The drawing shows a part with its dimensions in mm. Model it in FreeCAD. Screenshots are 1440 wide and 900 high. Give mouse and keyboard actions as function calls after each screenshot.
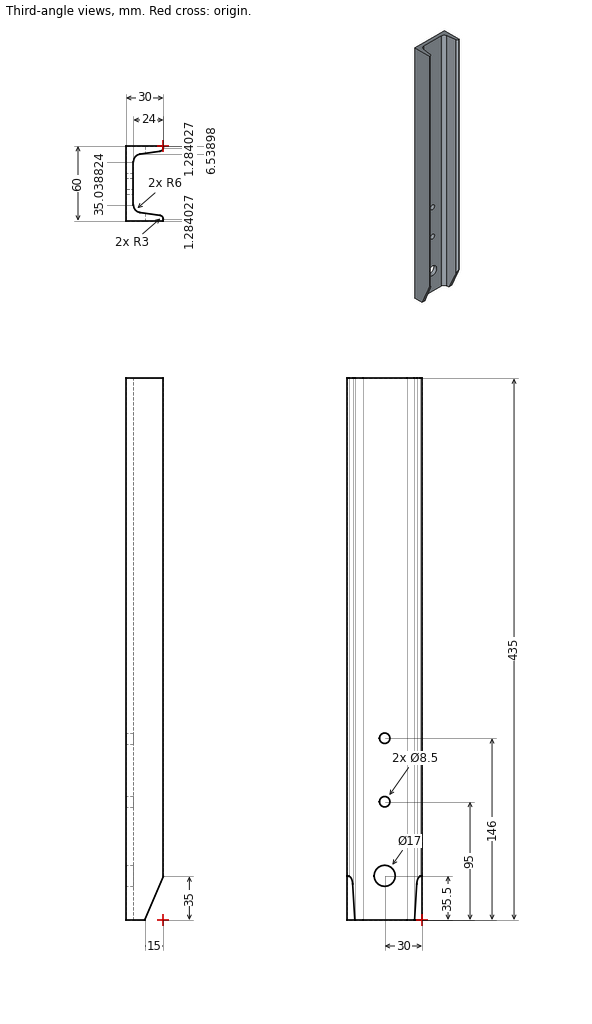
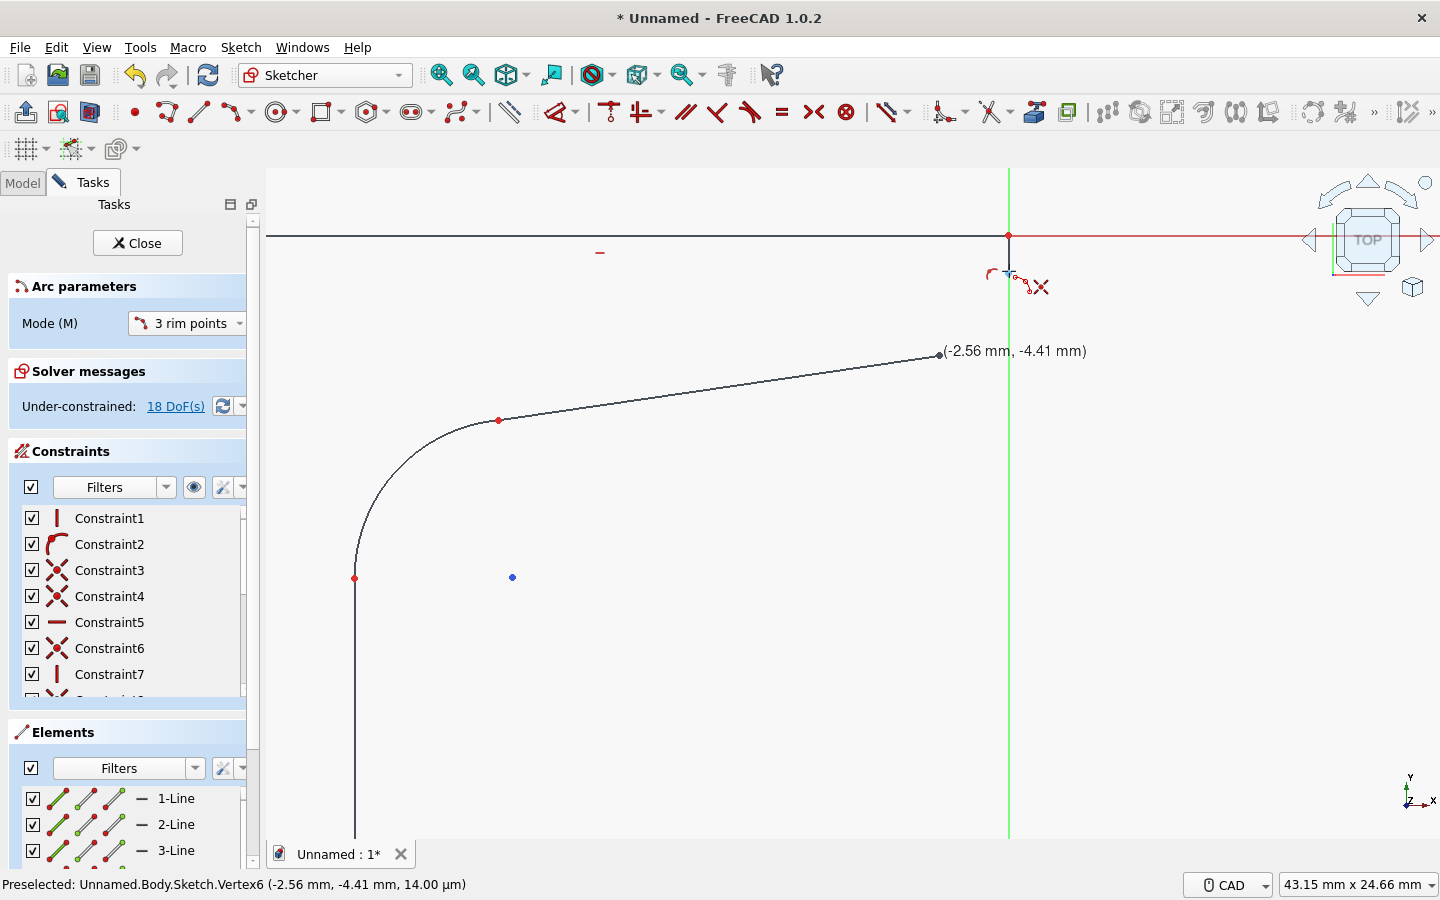
click(1009, 273)
click(989, 324)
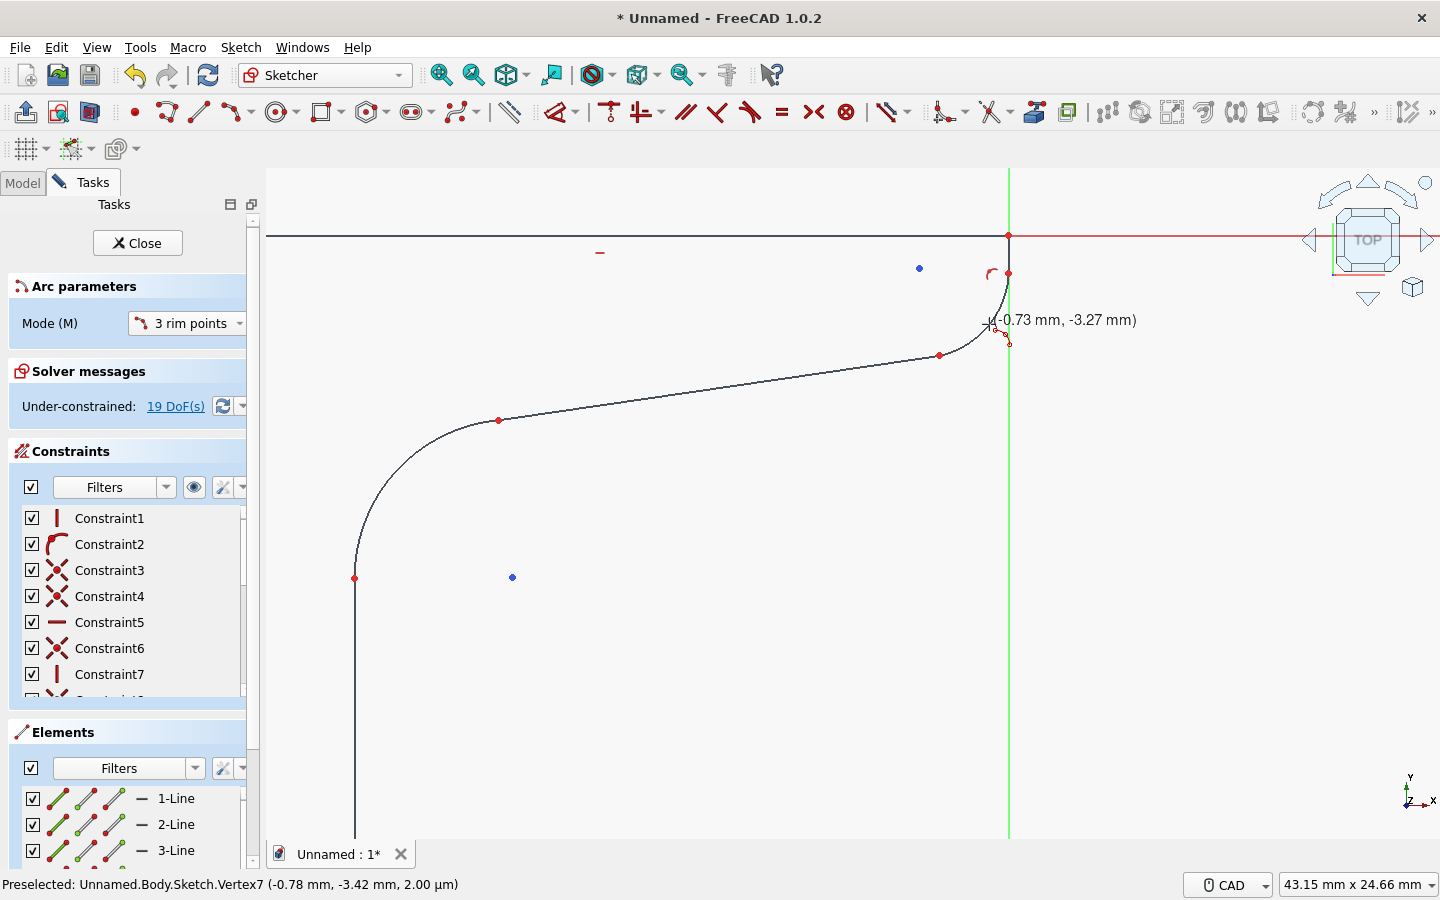
scroll(845, 324, down, 7)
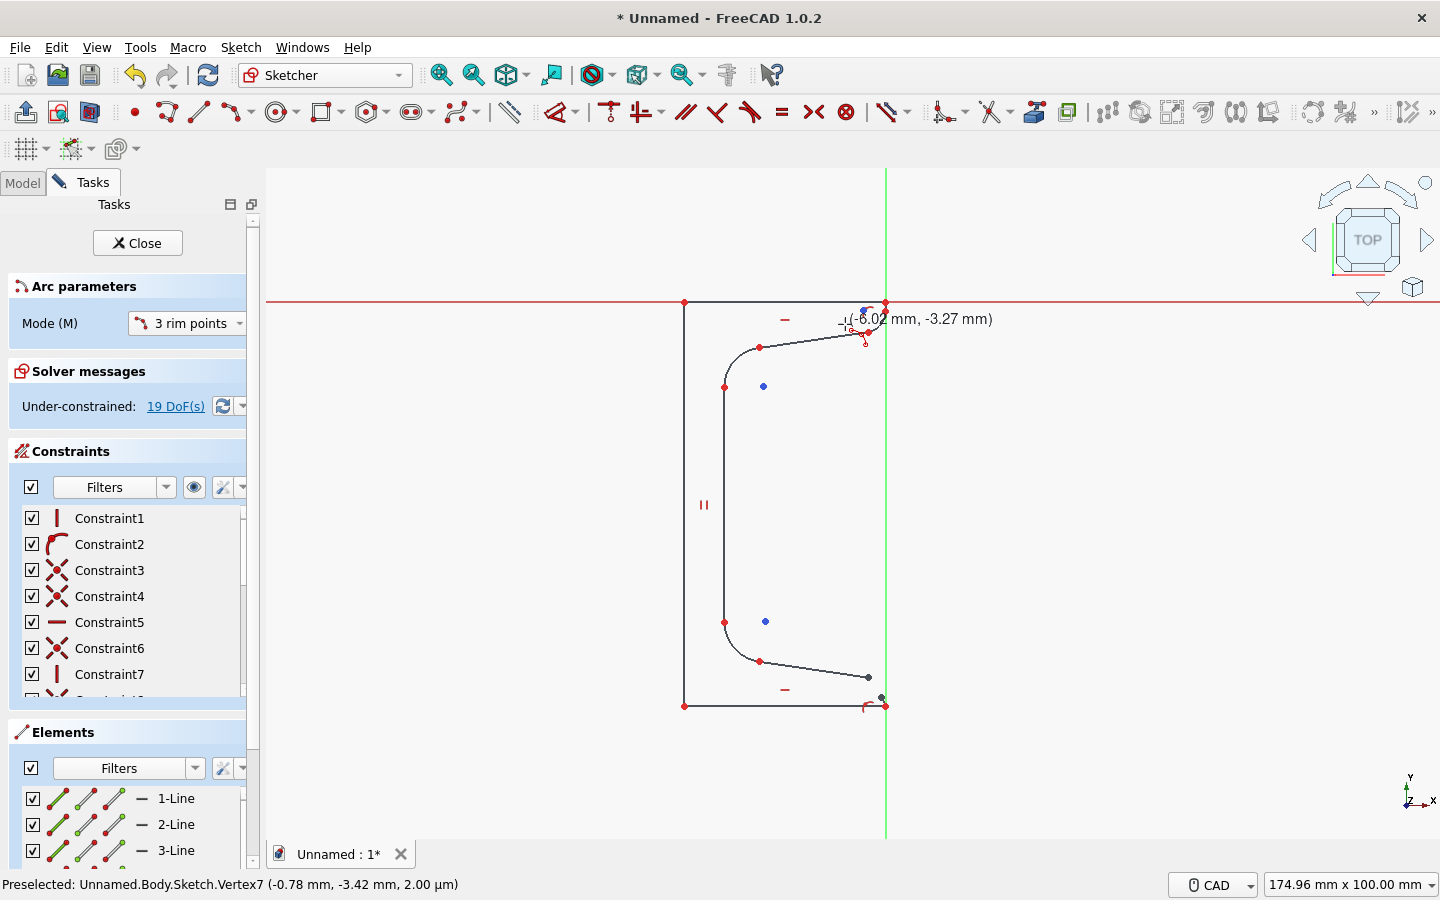
scroll(886, 696, up, 7)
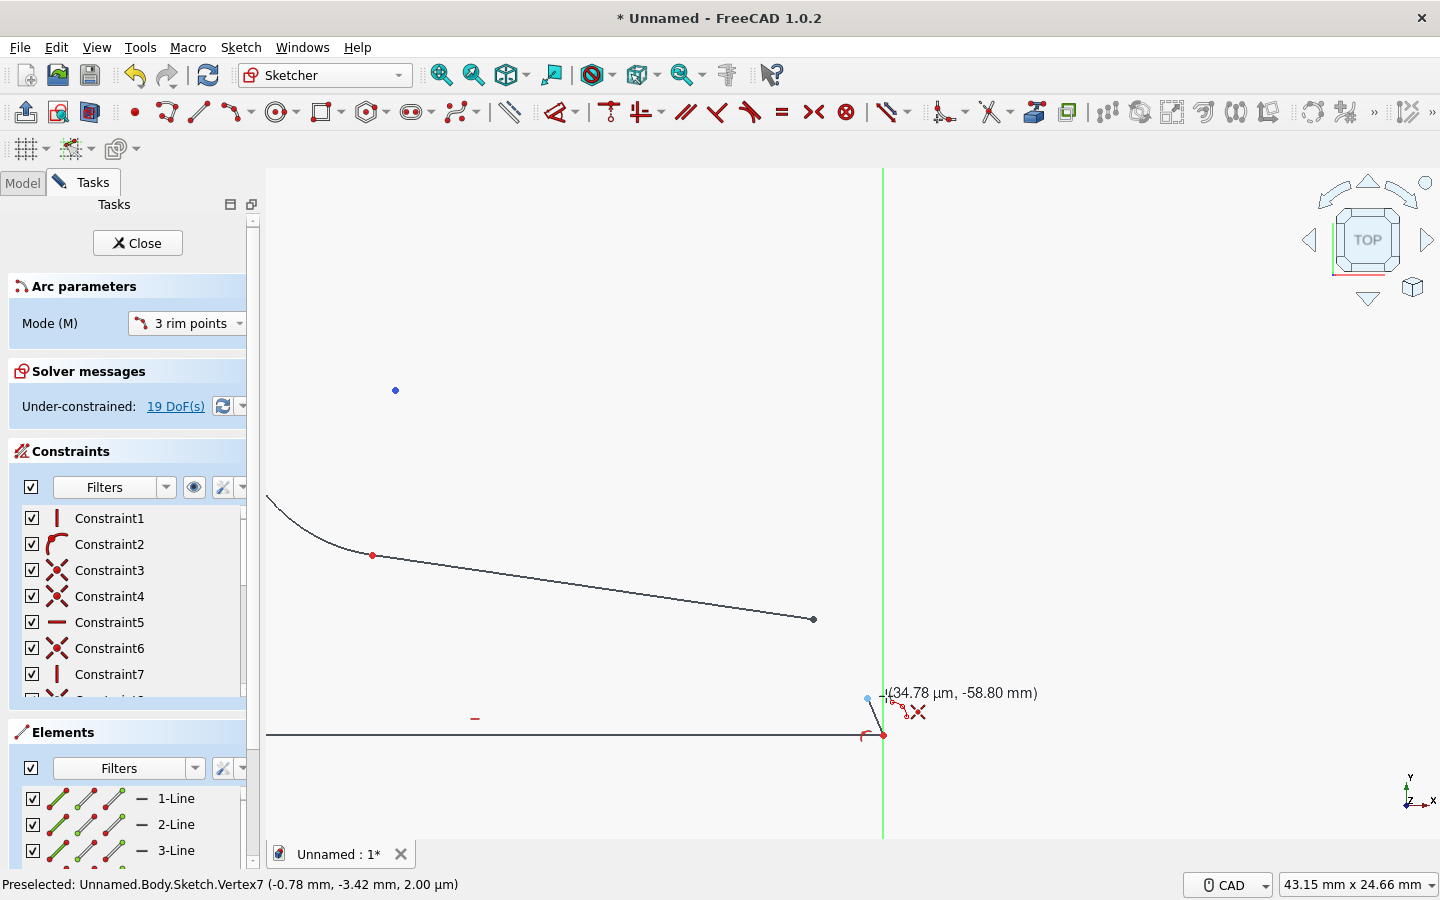
click(868, 698)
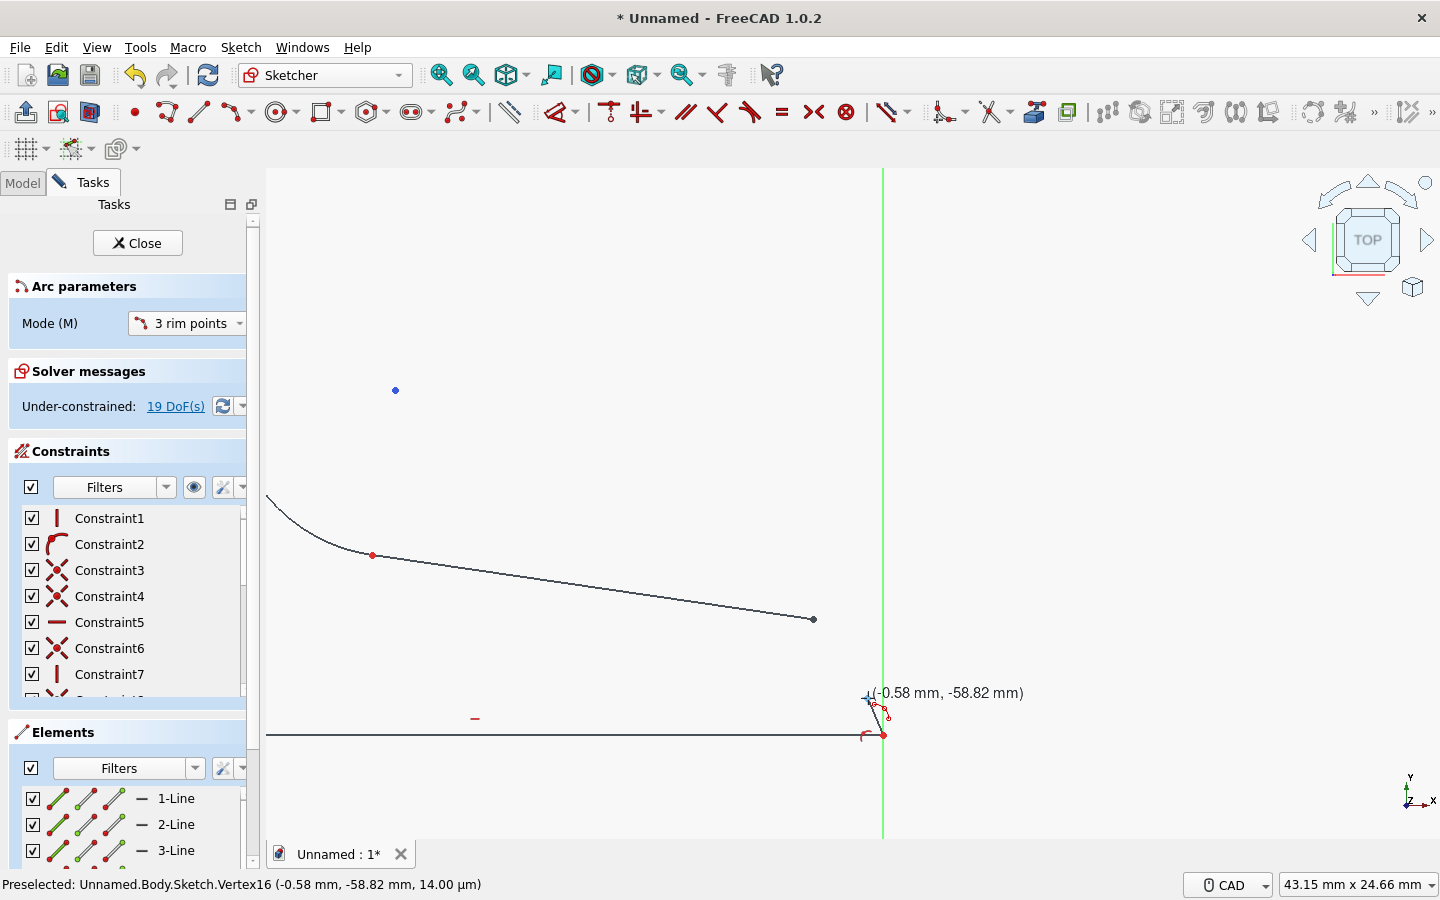
scroll(886, 696, down, 7)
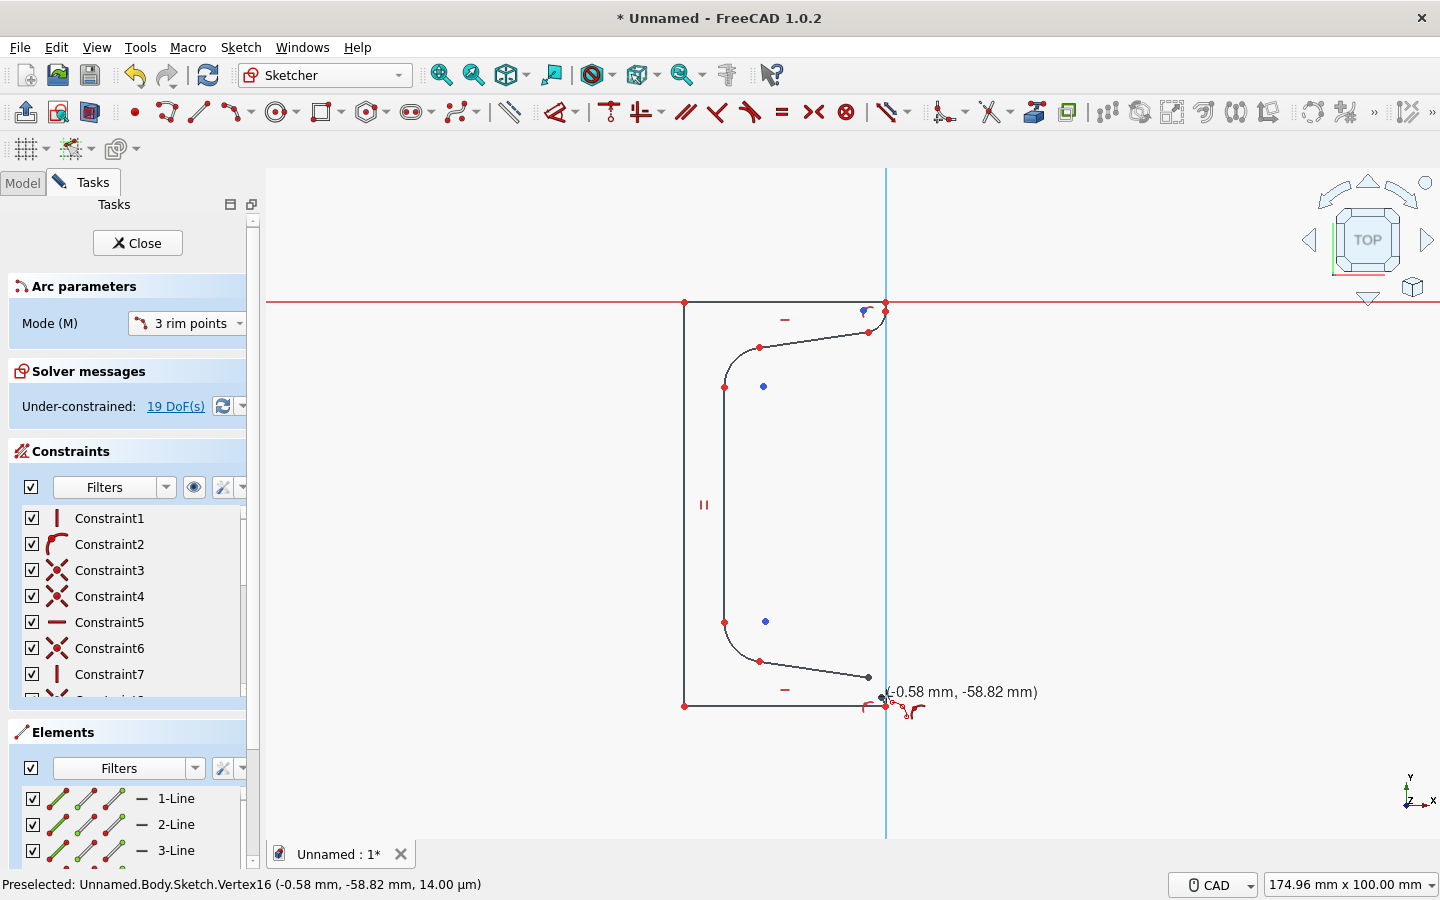
click(869, 678)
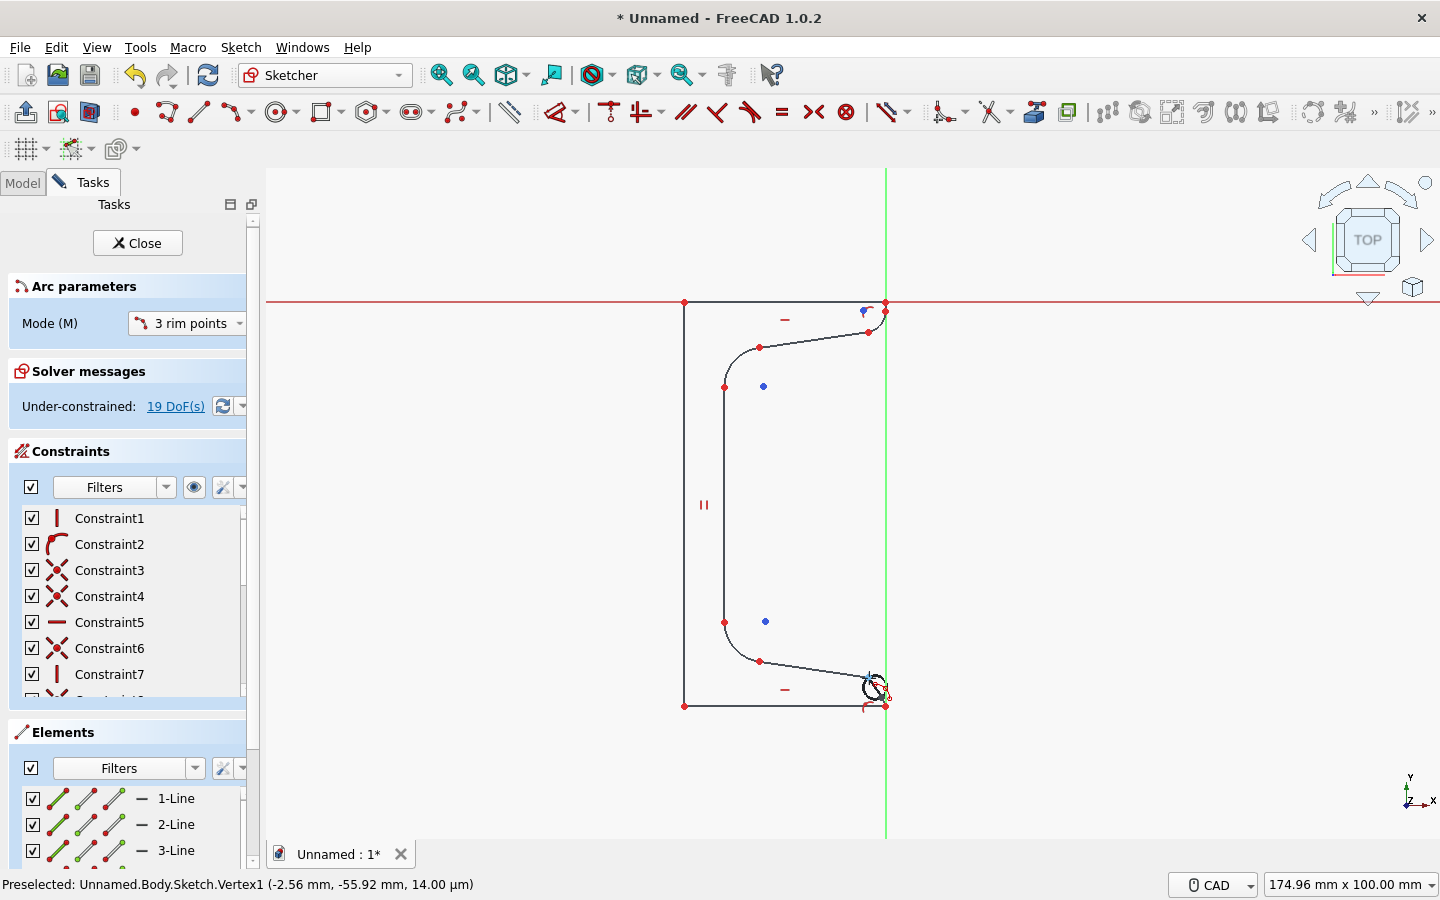
scroll(881, 683, up, 6)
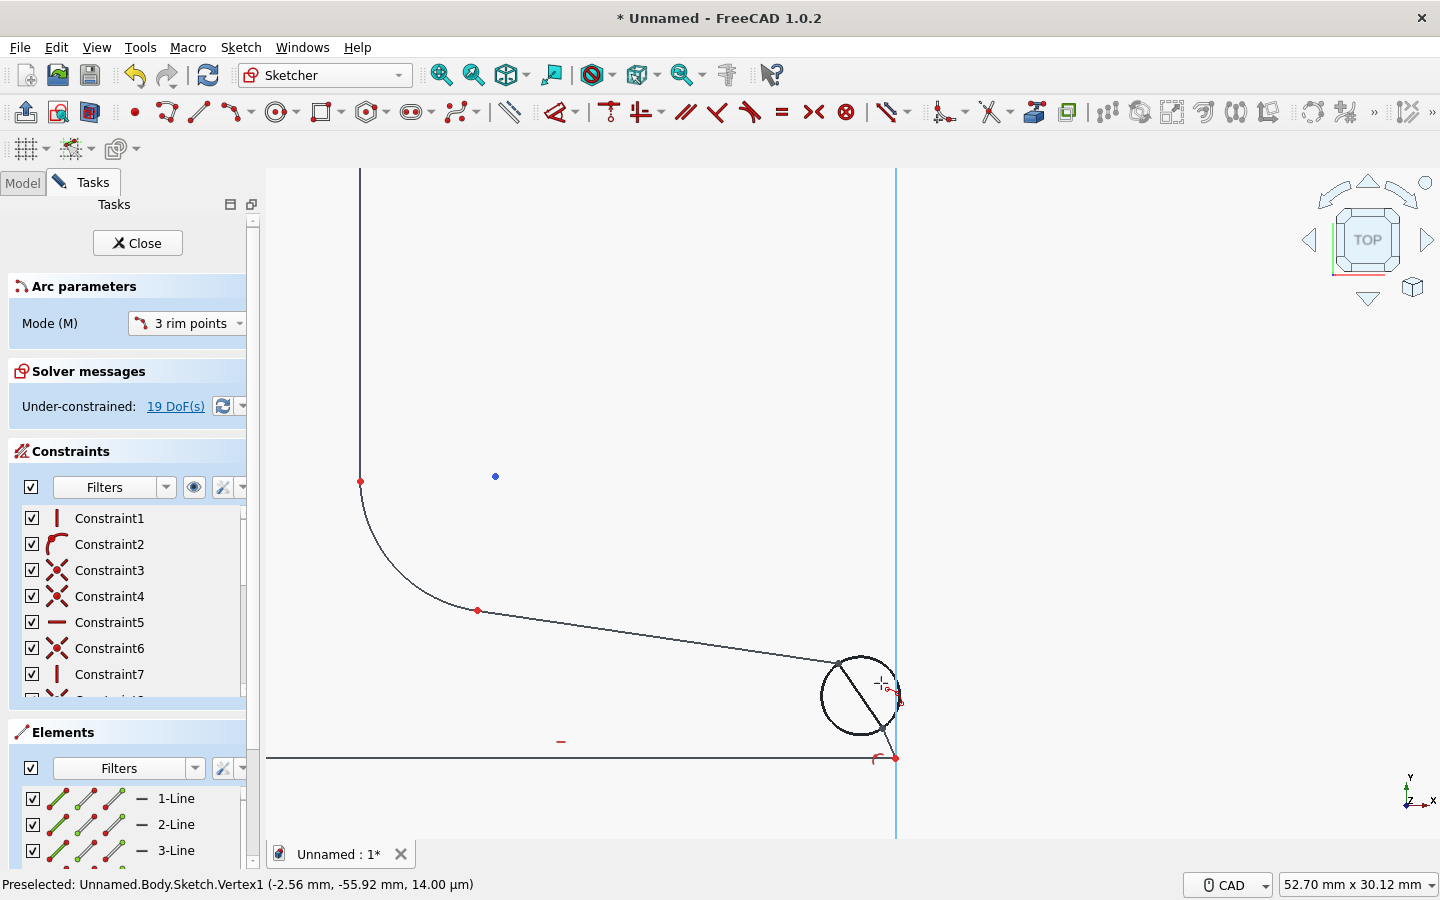
click(879, 682)
key(Escape)